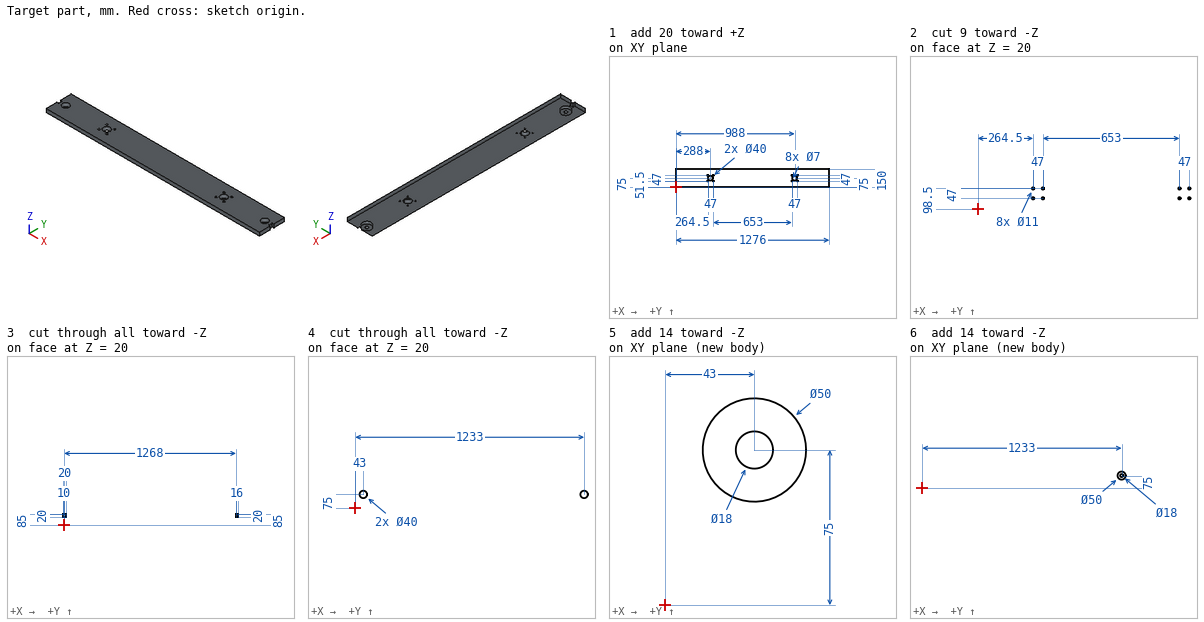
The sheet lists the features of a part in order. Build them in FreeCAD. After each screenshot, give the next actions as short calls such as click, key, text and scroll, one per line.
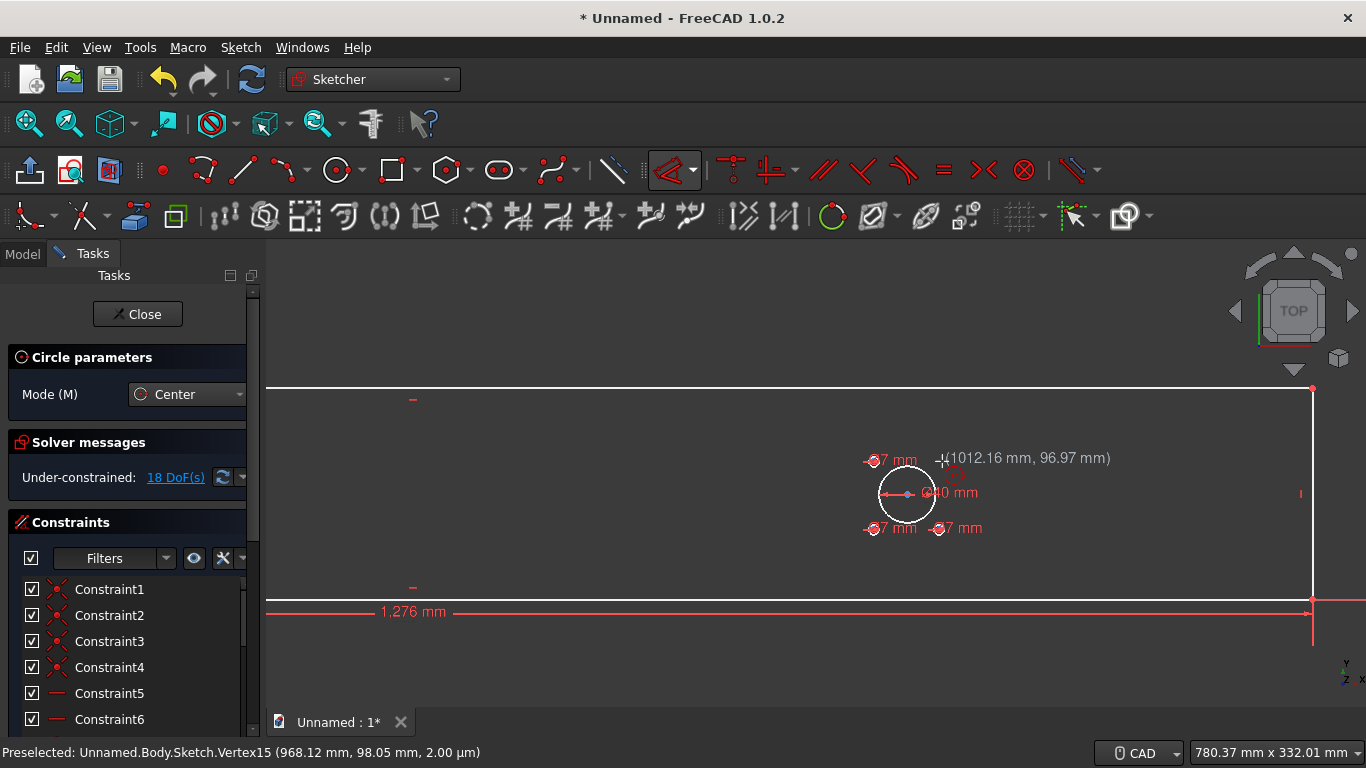
click(940, 461)
move(944, 457)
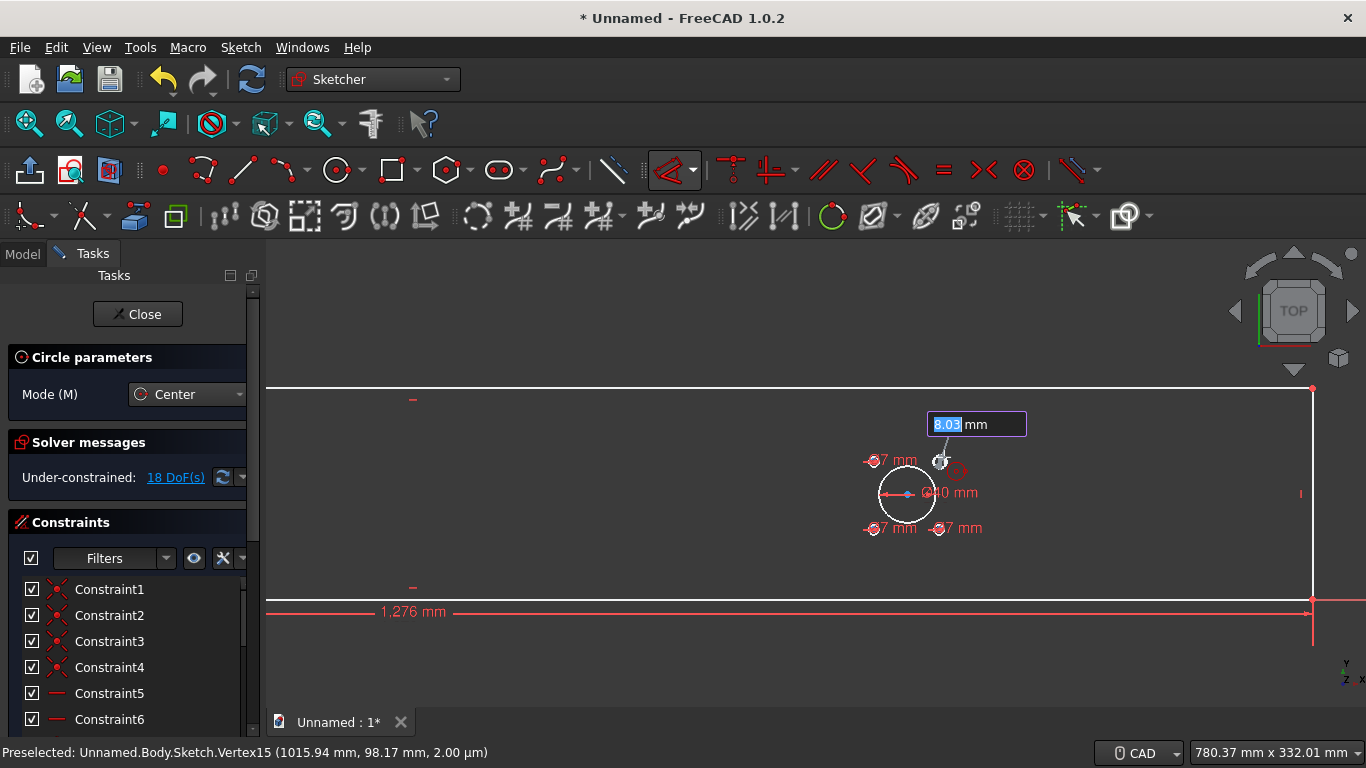
text(7)
key(Return)
key(Escape)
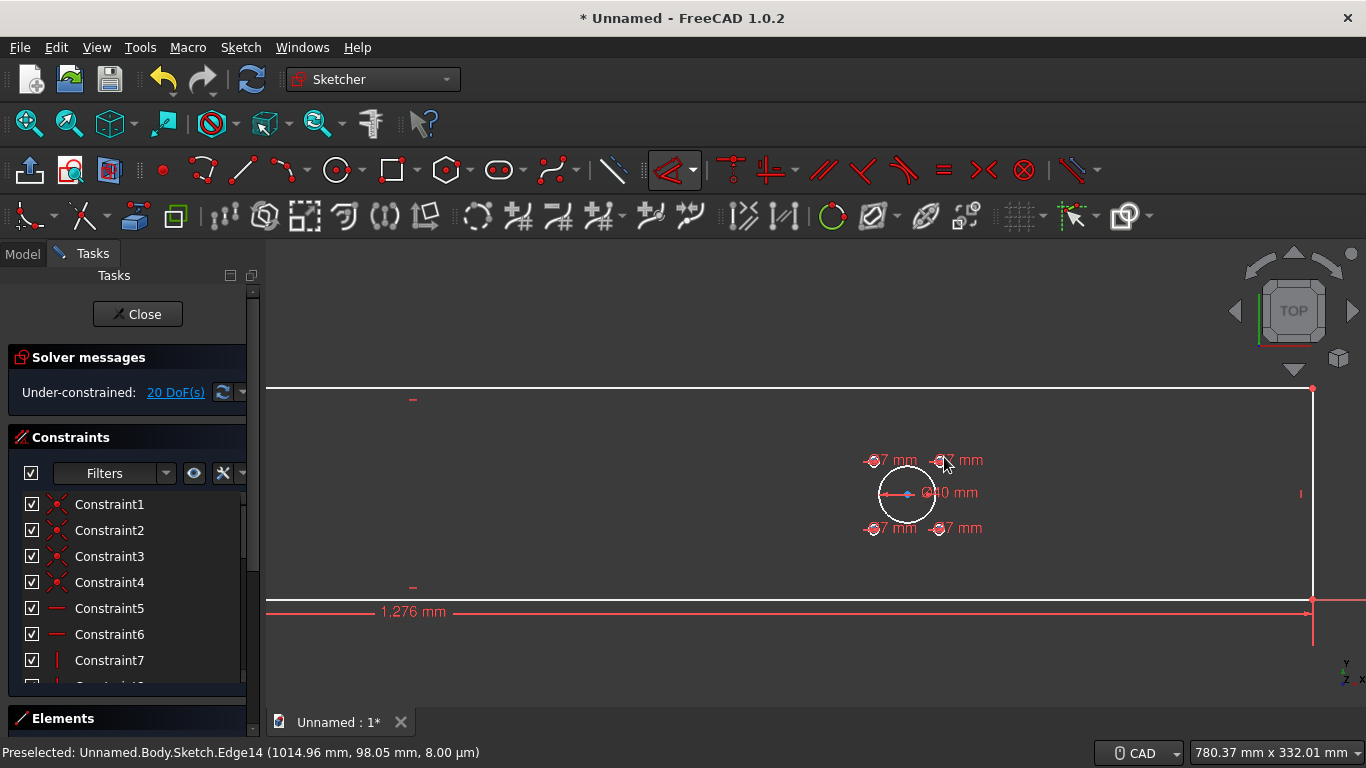
scroll(942, 461, down, 5)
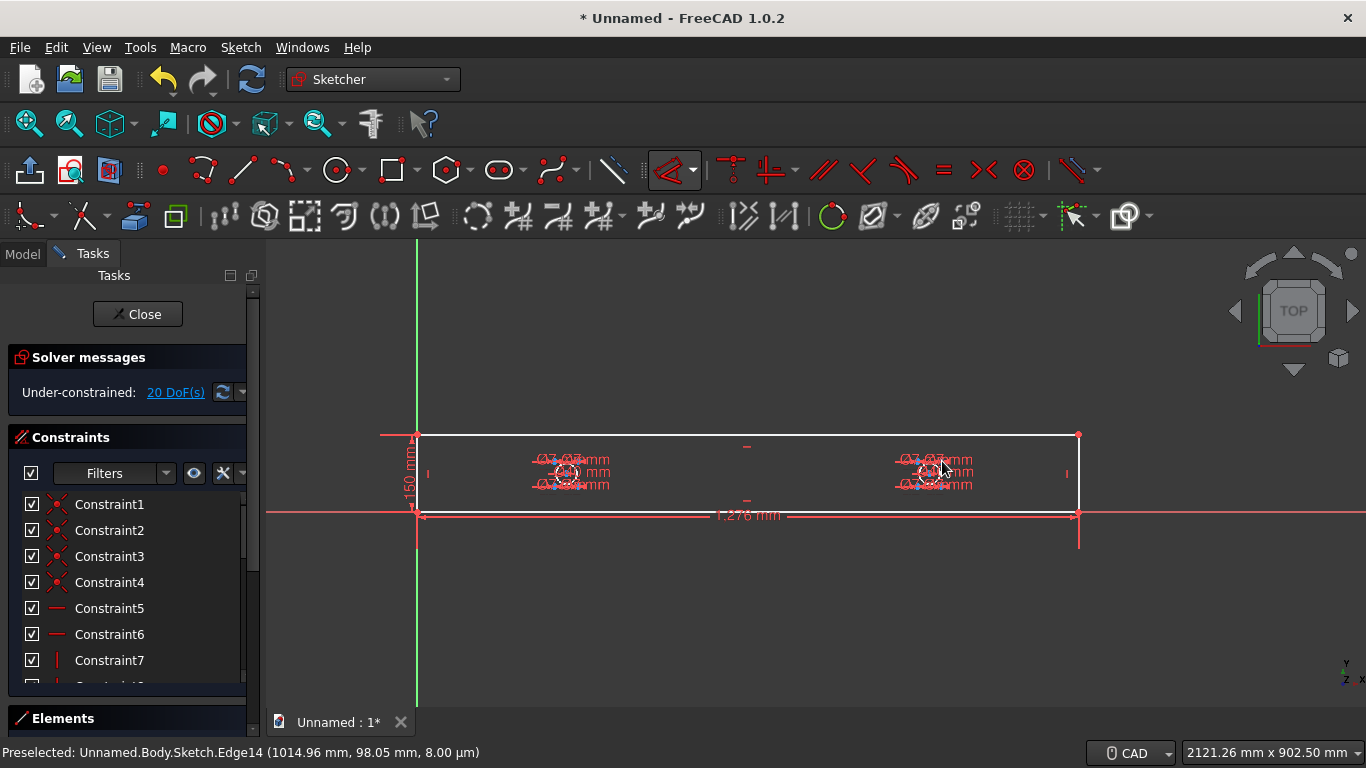
click(554, 487)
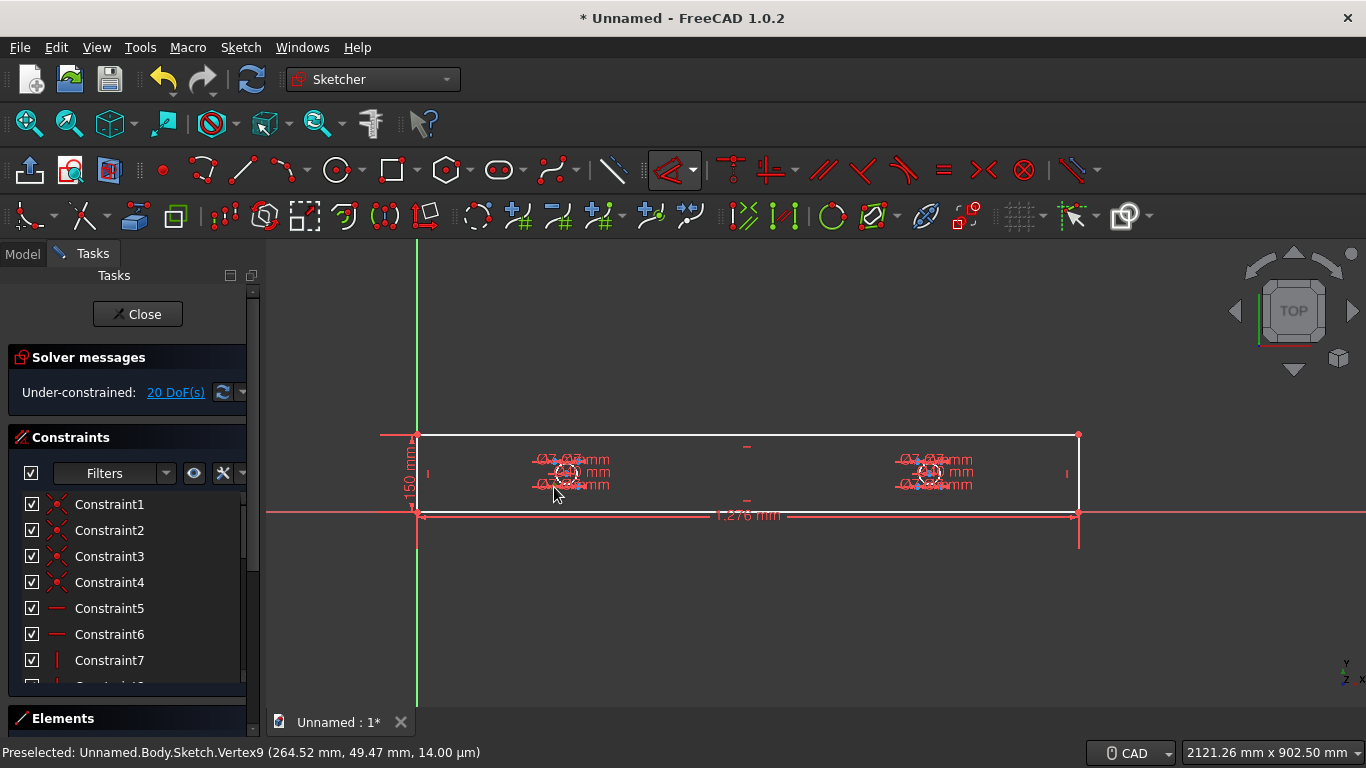
click(578, 487)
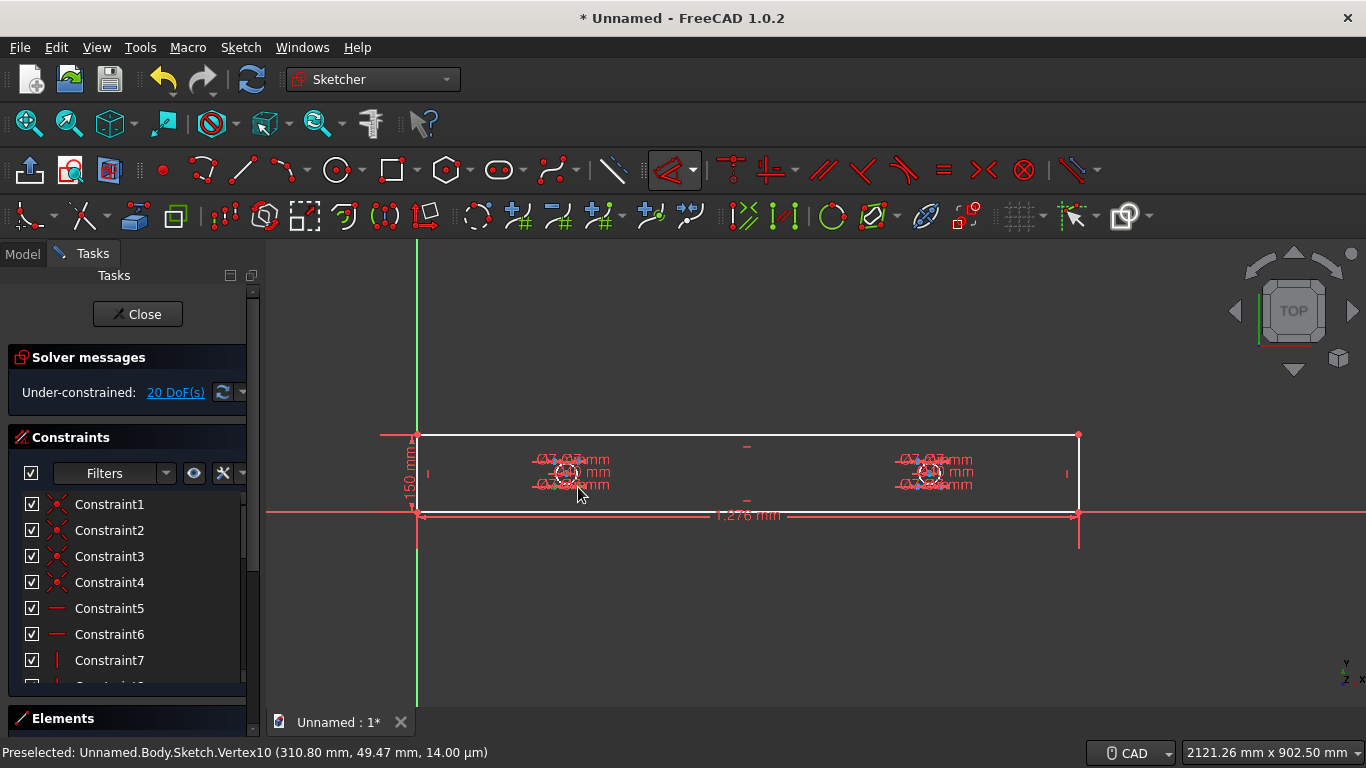
click(798, 170)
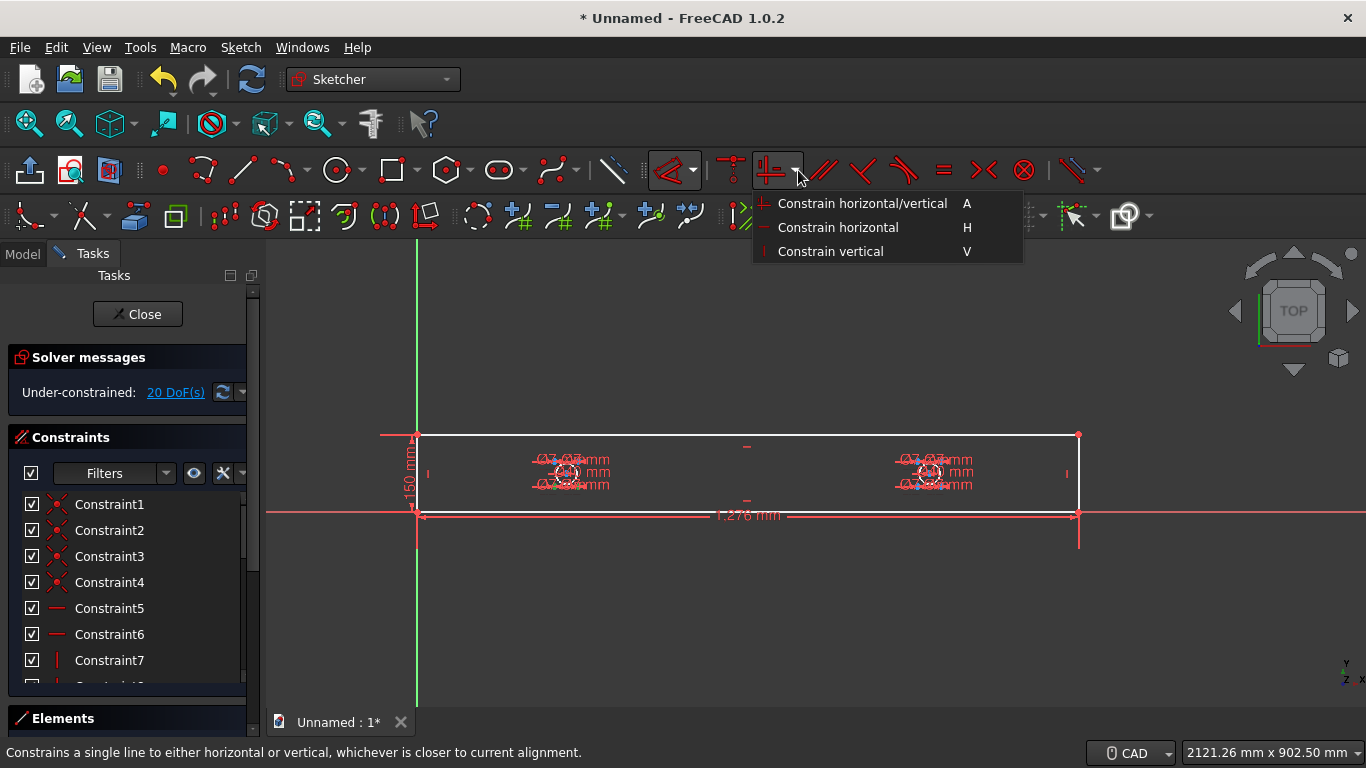
click(888, 227)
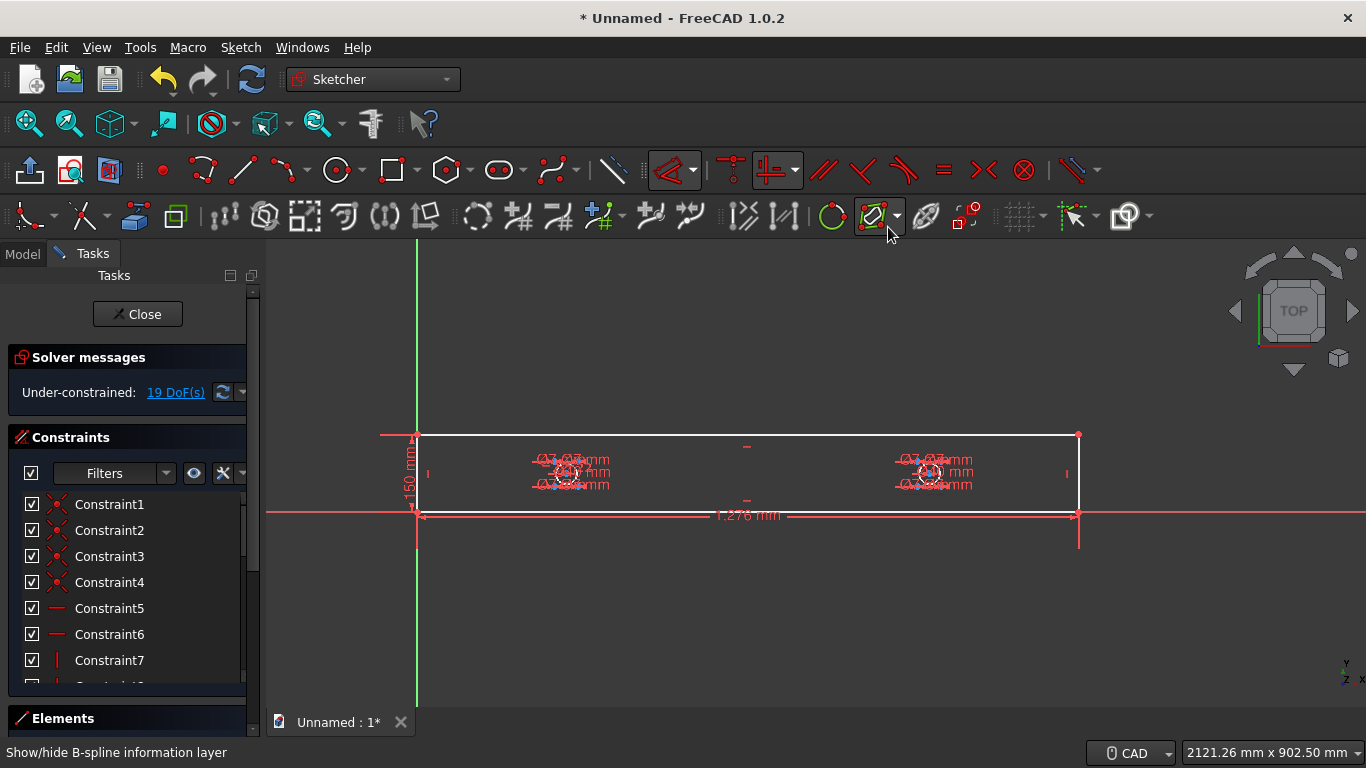
click(578, 487)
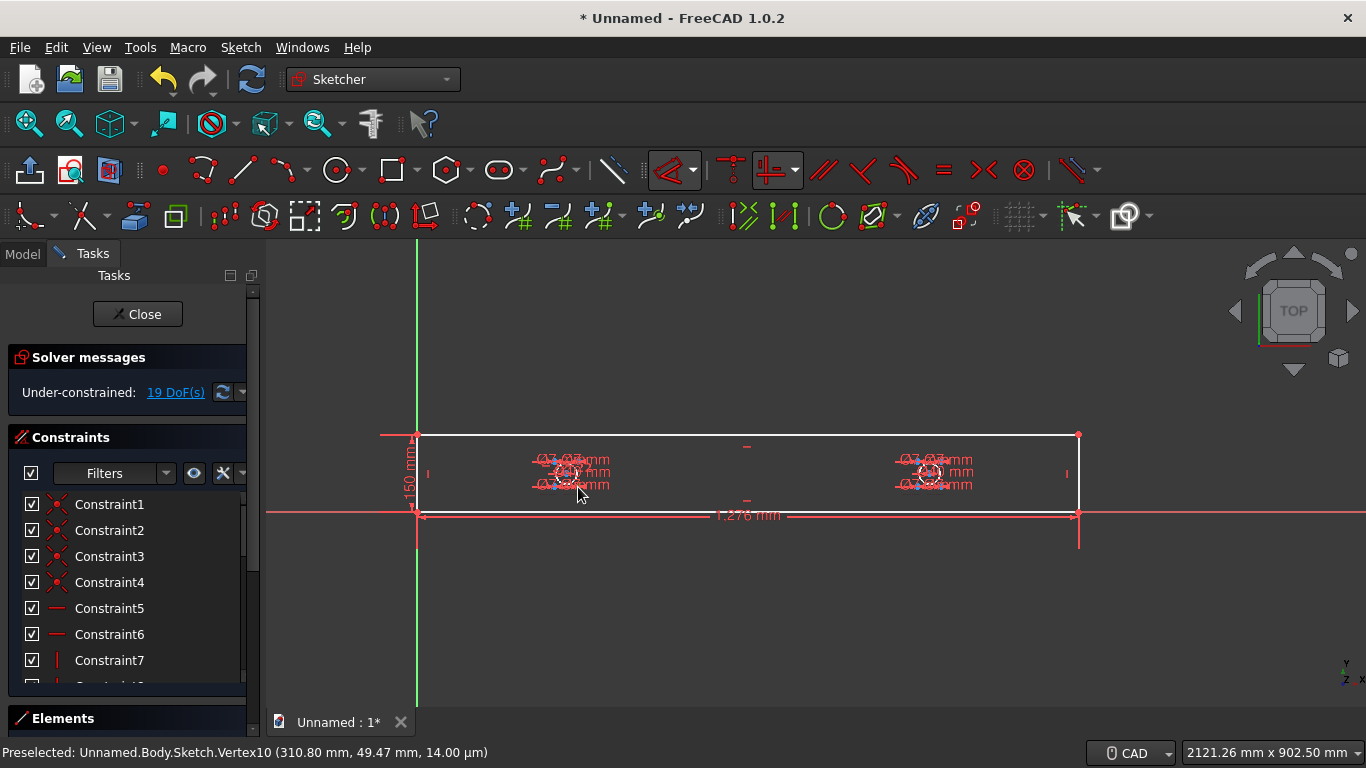
click(917, 487)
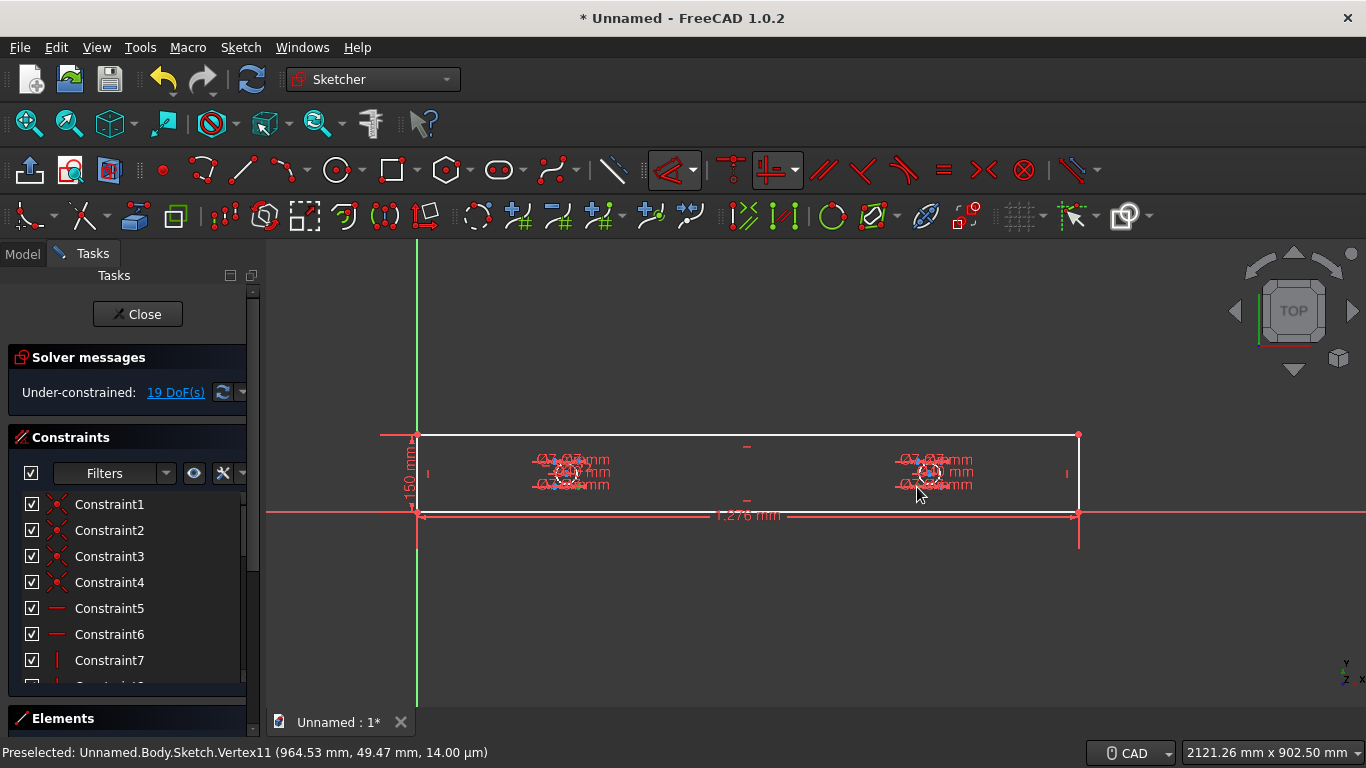
click(798, 170)